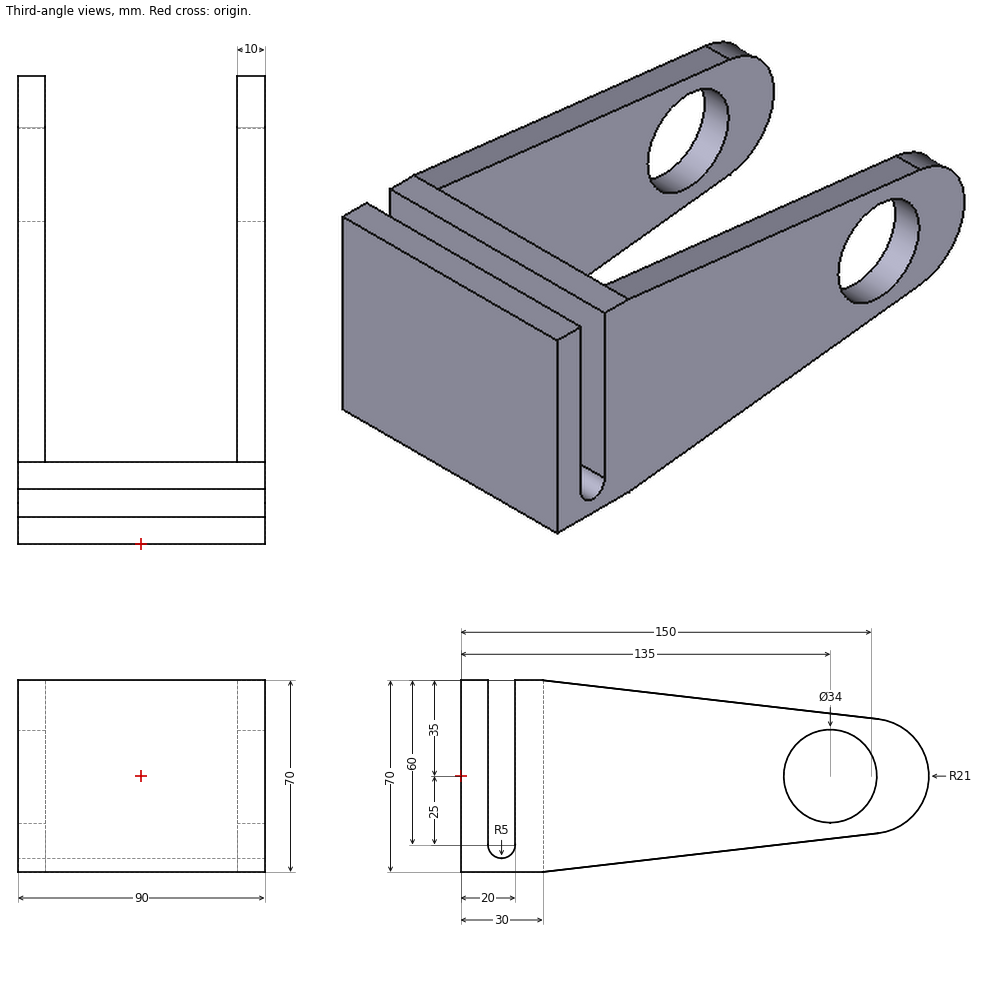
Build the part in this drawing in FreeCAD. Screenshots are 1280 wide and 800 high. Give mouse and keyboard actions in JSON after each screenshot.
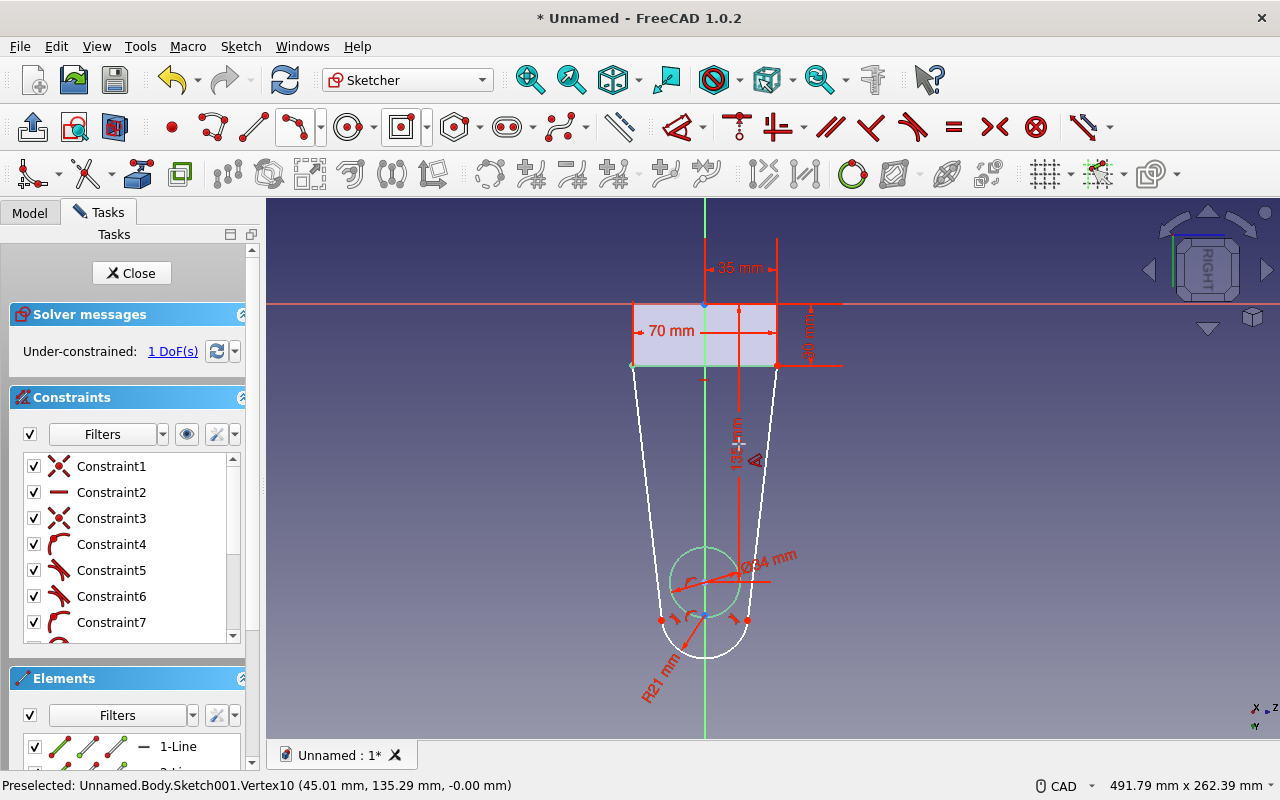
{"action": "left_click", "coordinate": [705, 615]}
{"action": "left_click", "coordinate": [739, 388]}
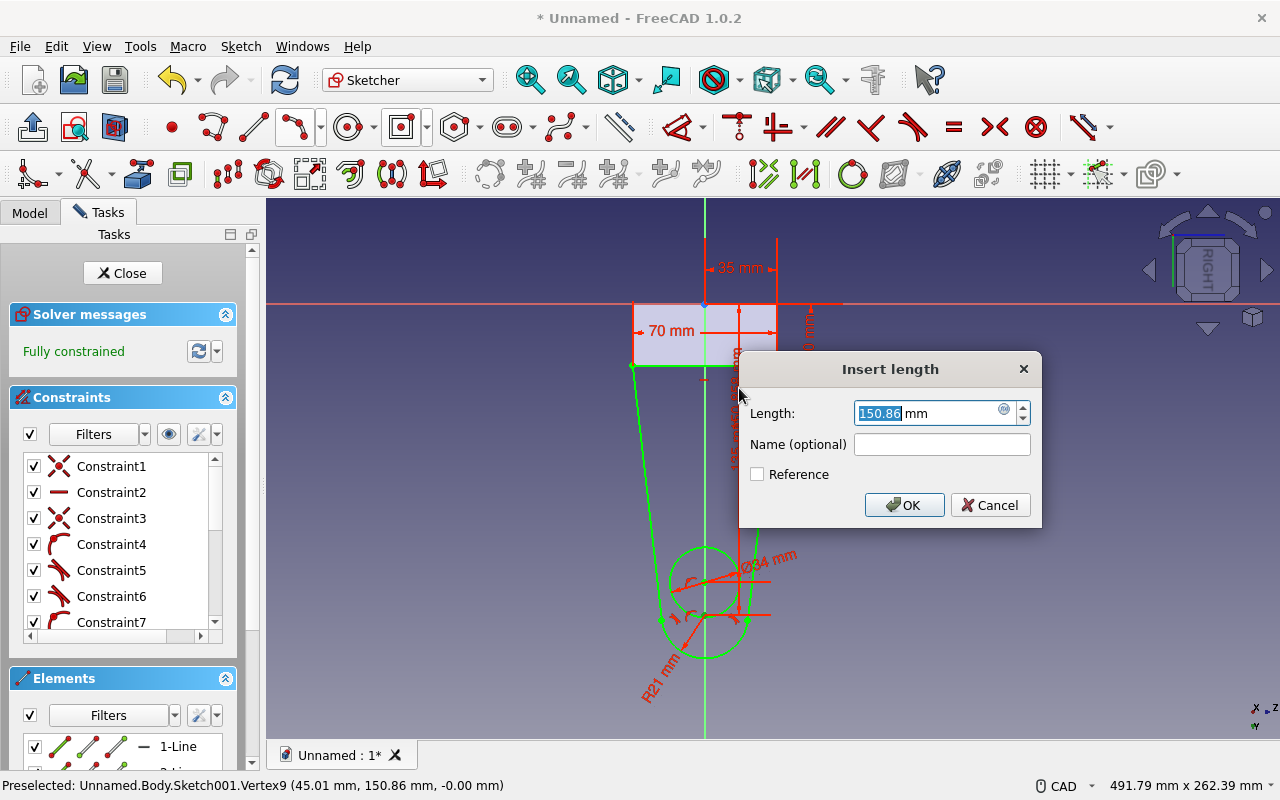
{"action": "type", "text": "150"}
{"action": "key", "text": "Return"}
{"action": "key", "text": "Escape"}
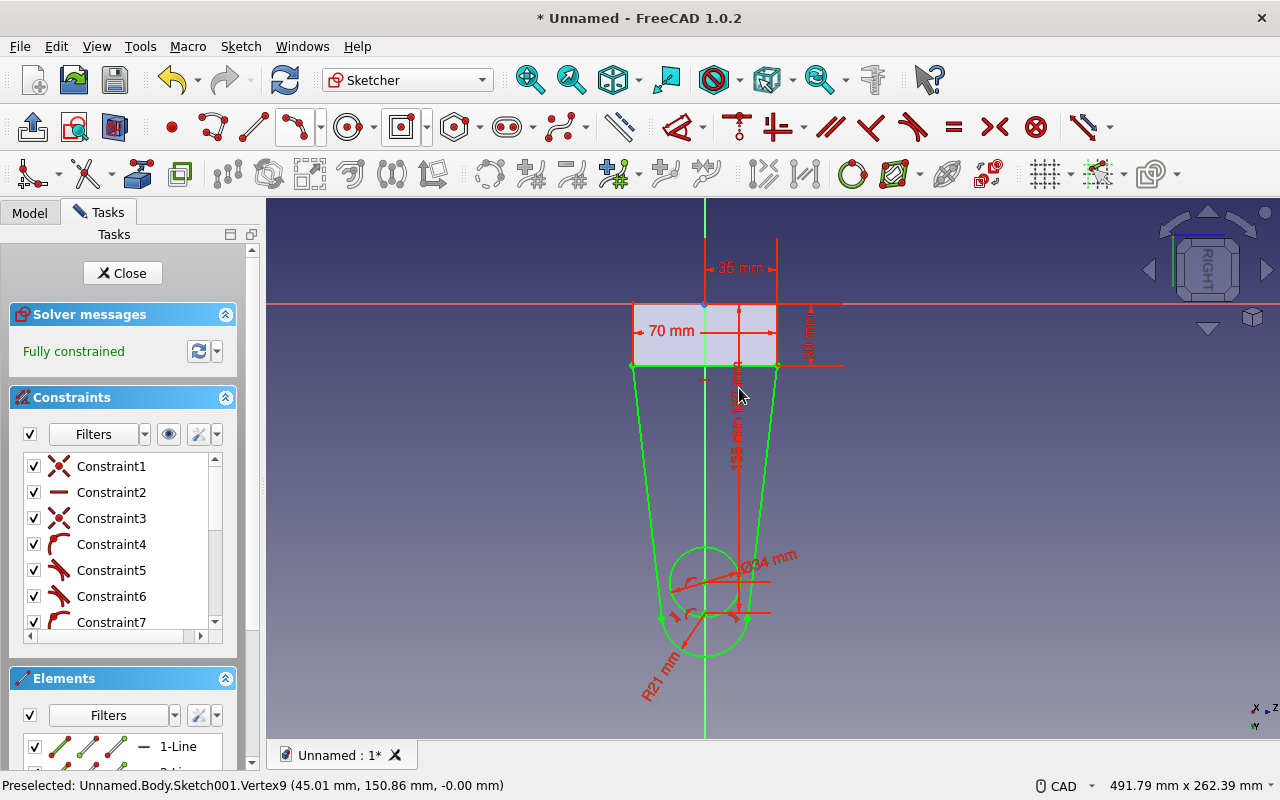
{"action": "left_click", "coordinate": [123, 273]}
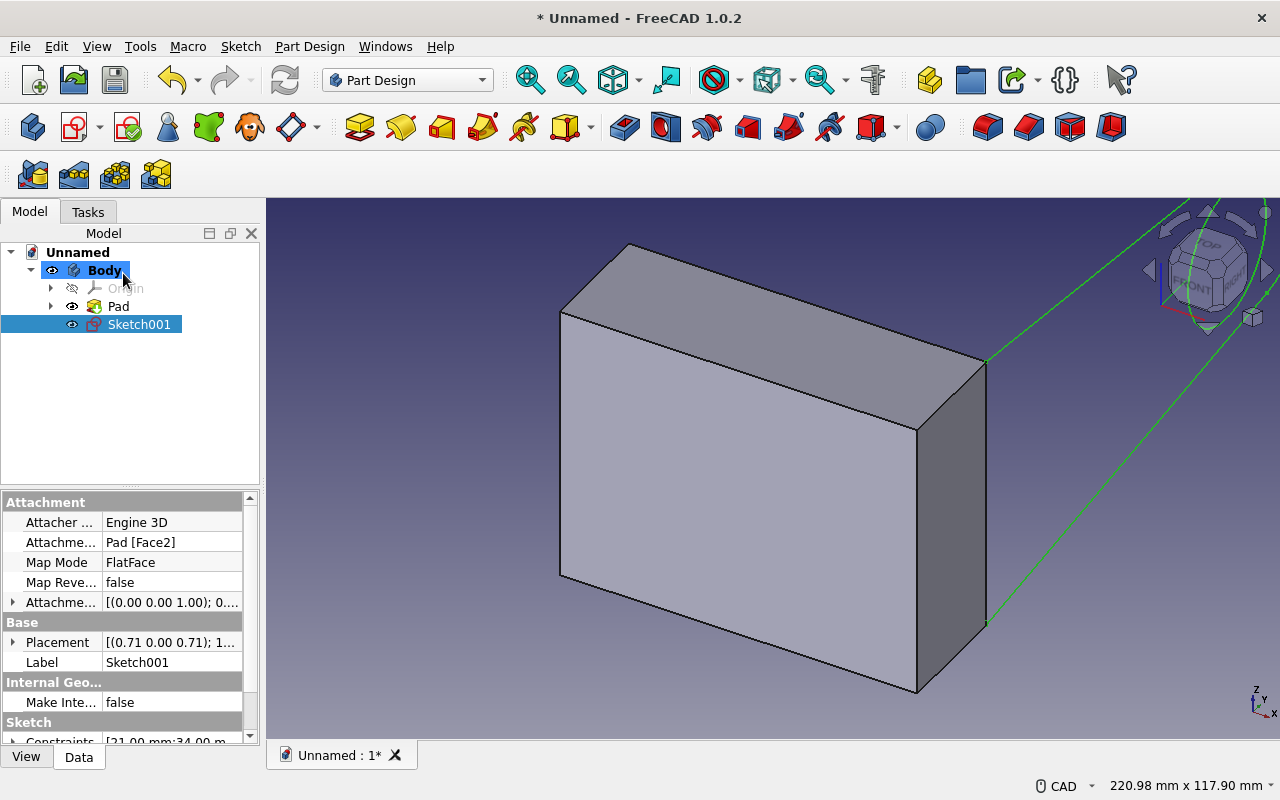
{"action": "left_click", "coordinate": [360, 128]}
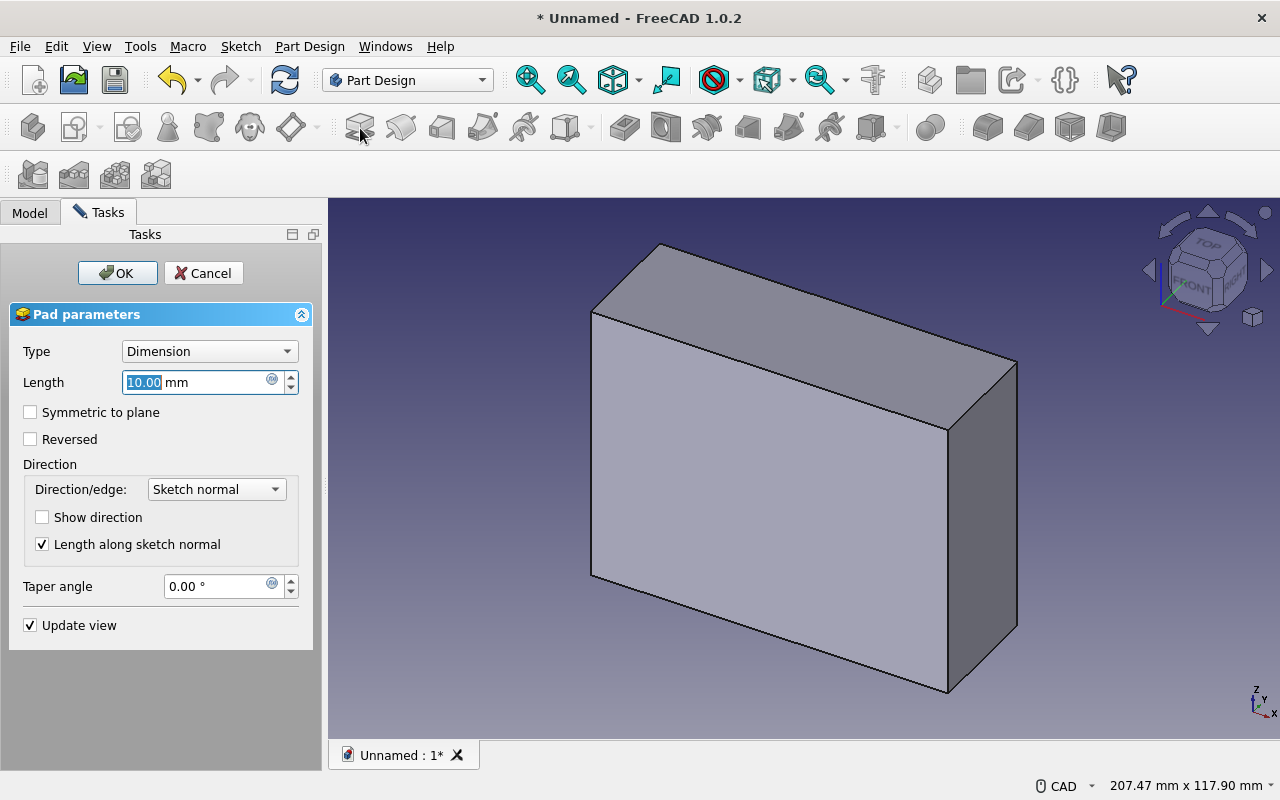
{"action": "type", "text": "10"}
{"action": "key", "text": "Tab"}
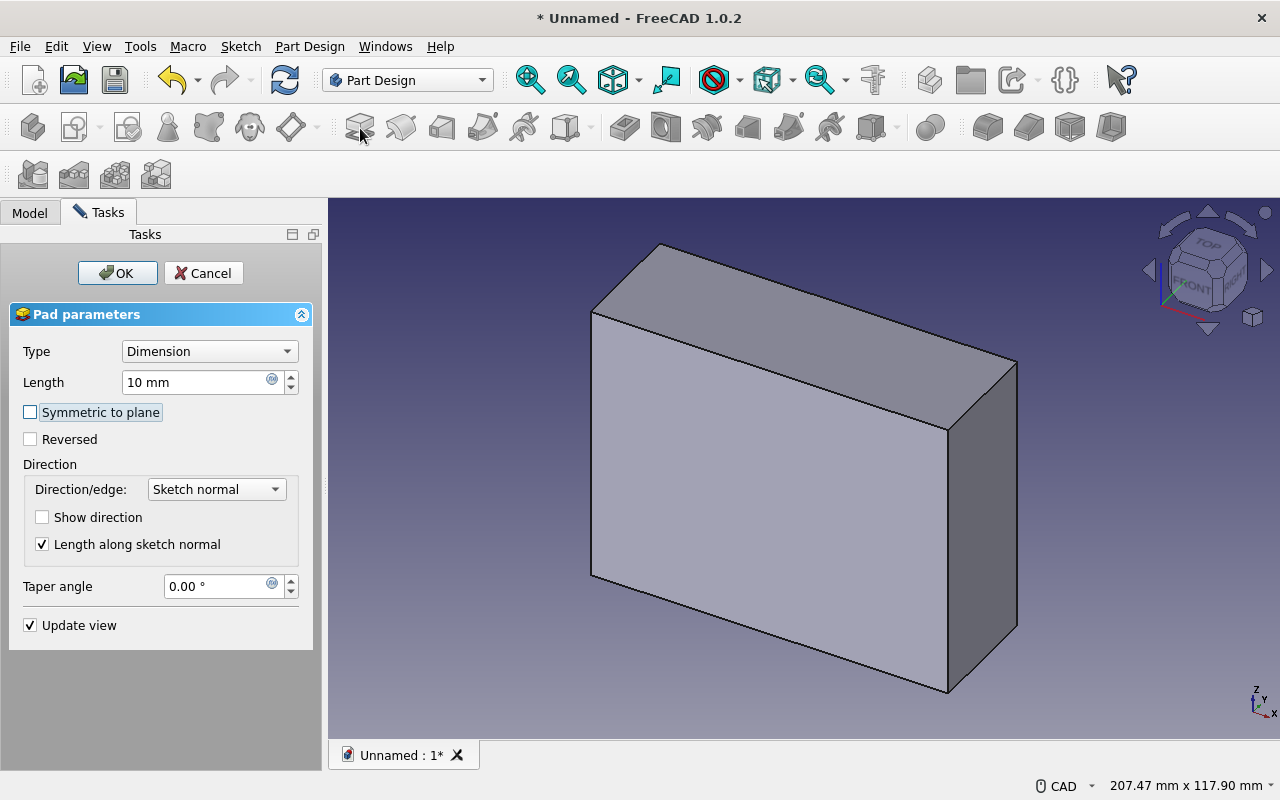
{"action": "left_click", "coordinate": [31, 439]}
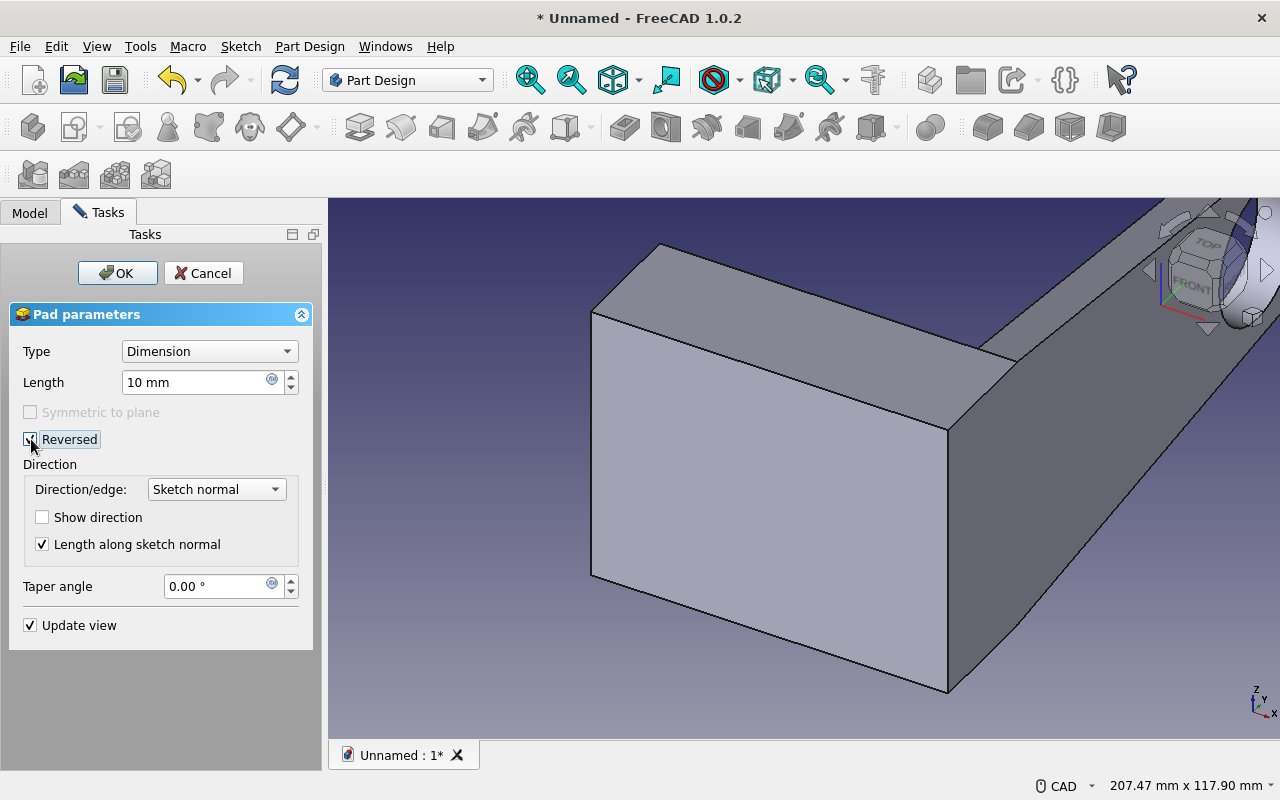
{"action": "left_click", "coordinate": [118, 273]}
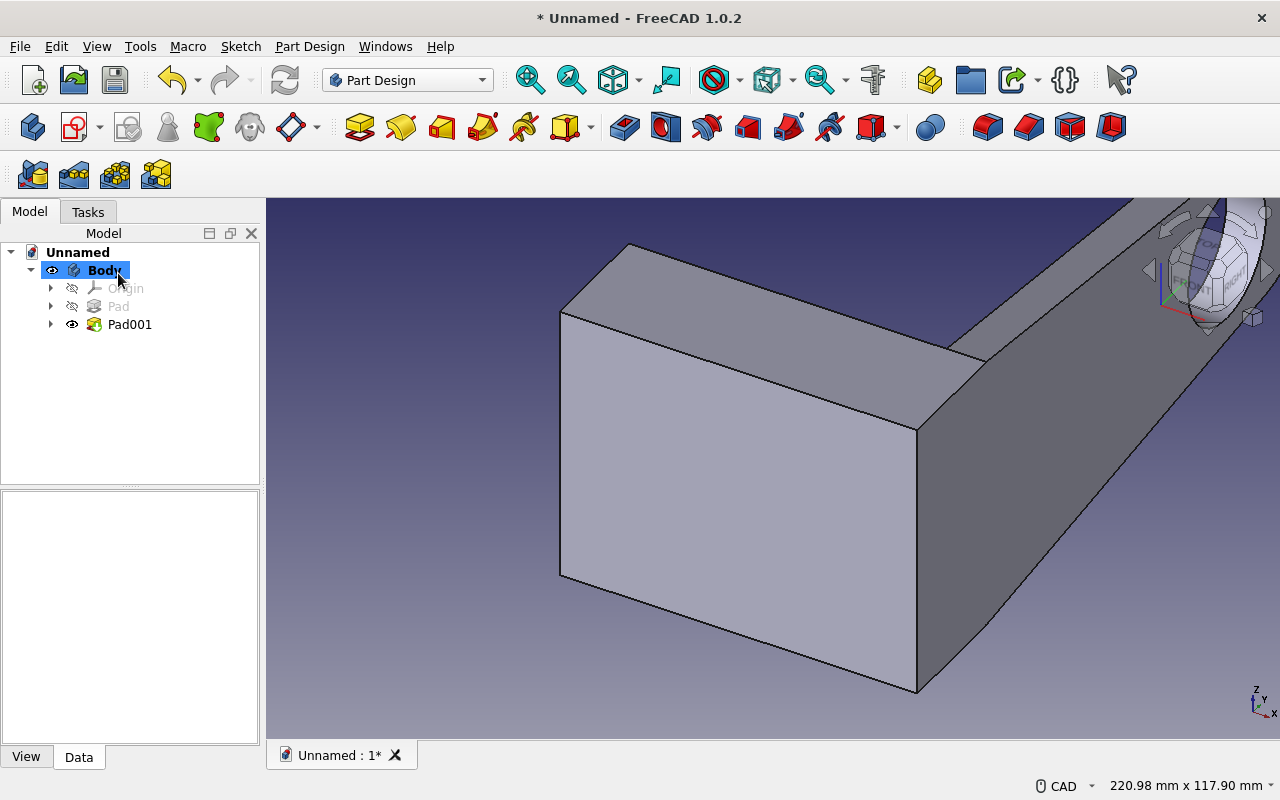
{"action": "left_click", "coordinate": [531, 80]}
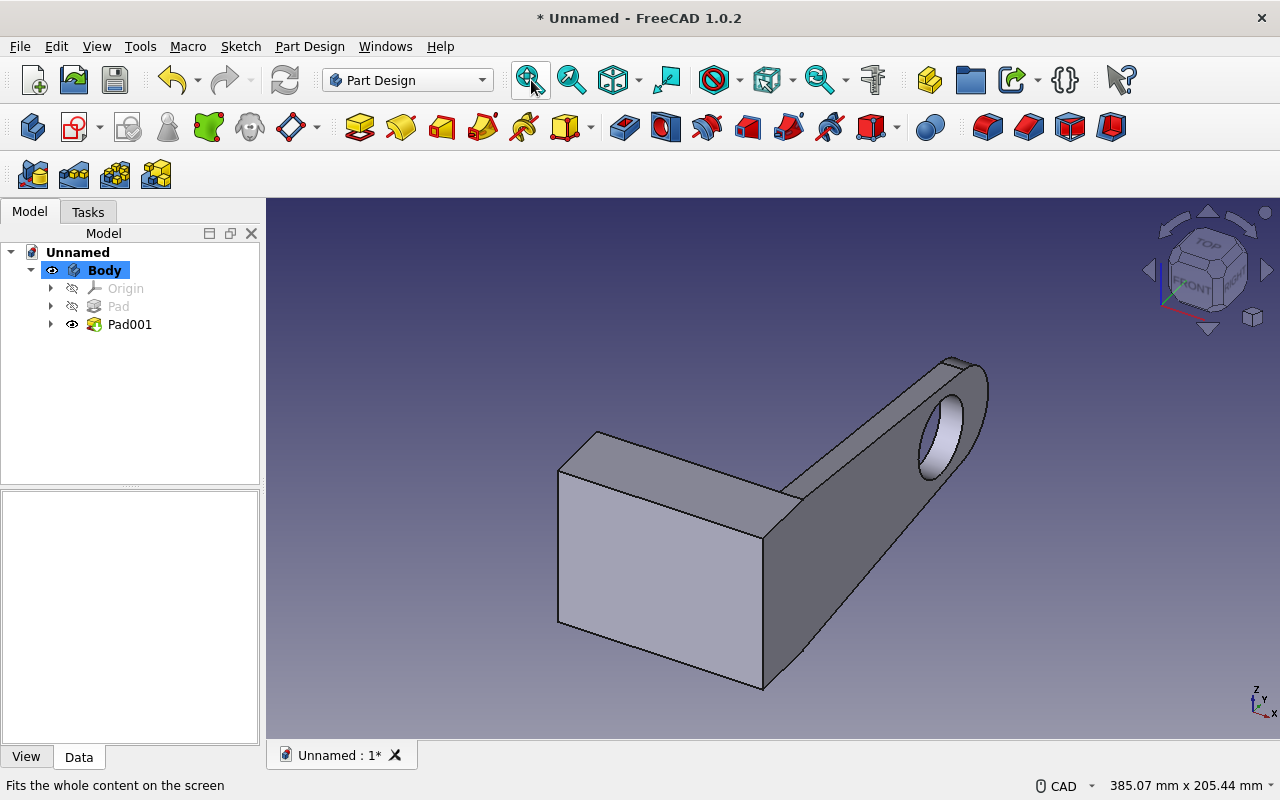
{"action": "left_click", "coordinate": [117, 324]}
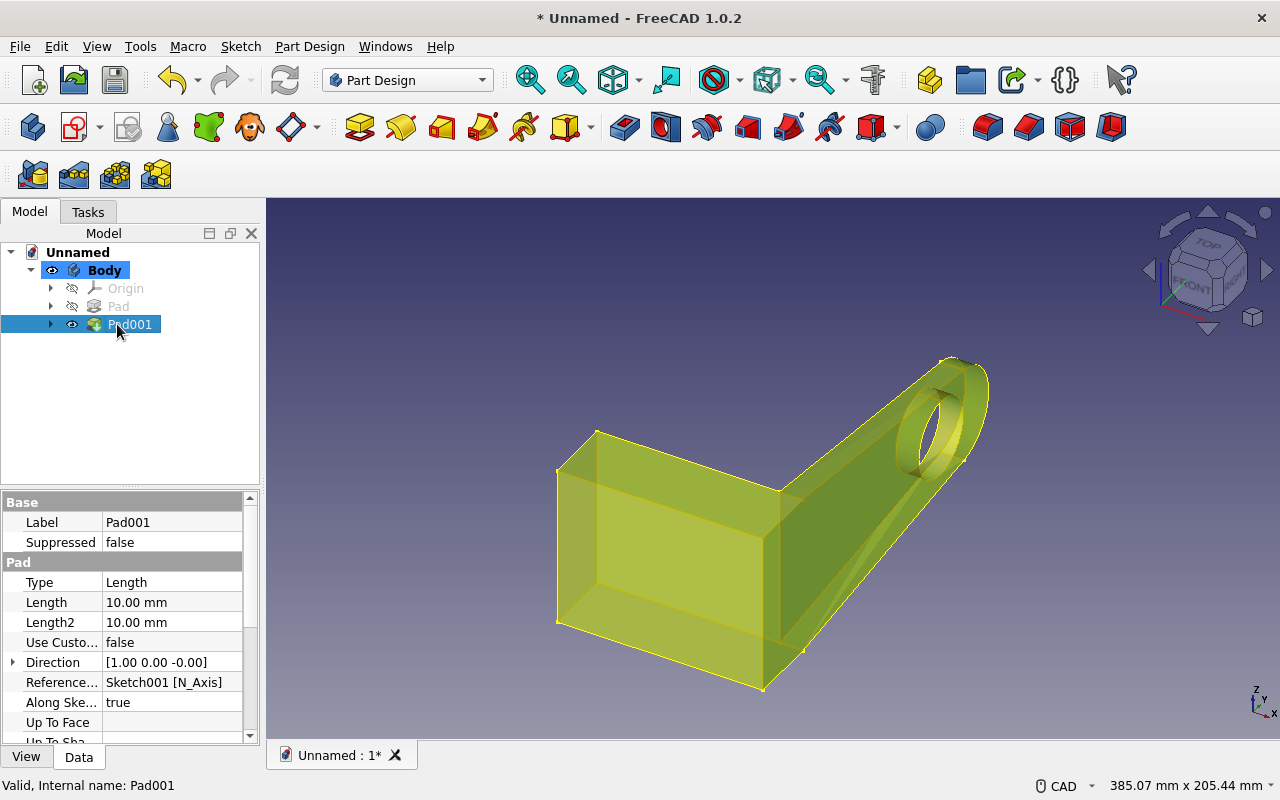
{"action": "left_click", "coordinate": [33, 174]}